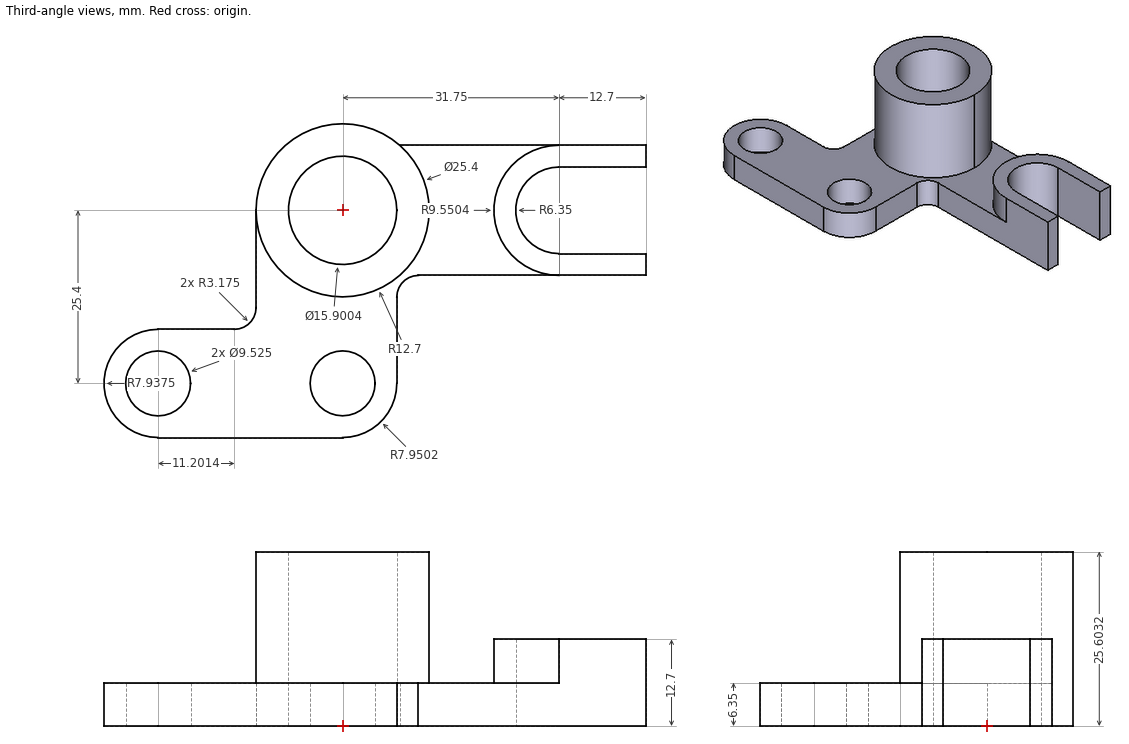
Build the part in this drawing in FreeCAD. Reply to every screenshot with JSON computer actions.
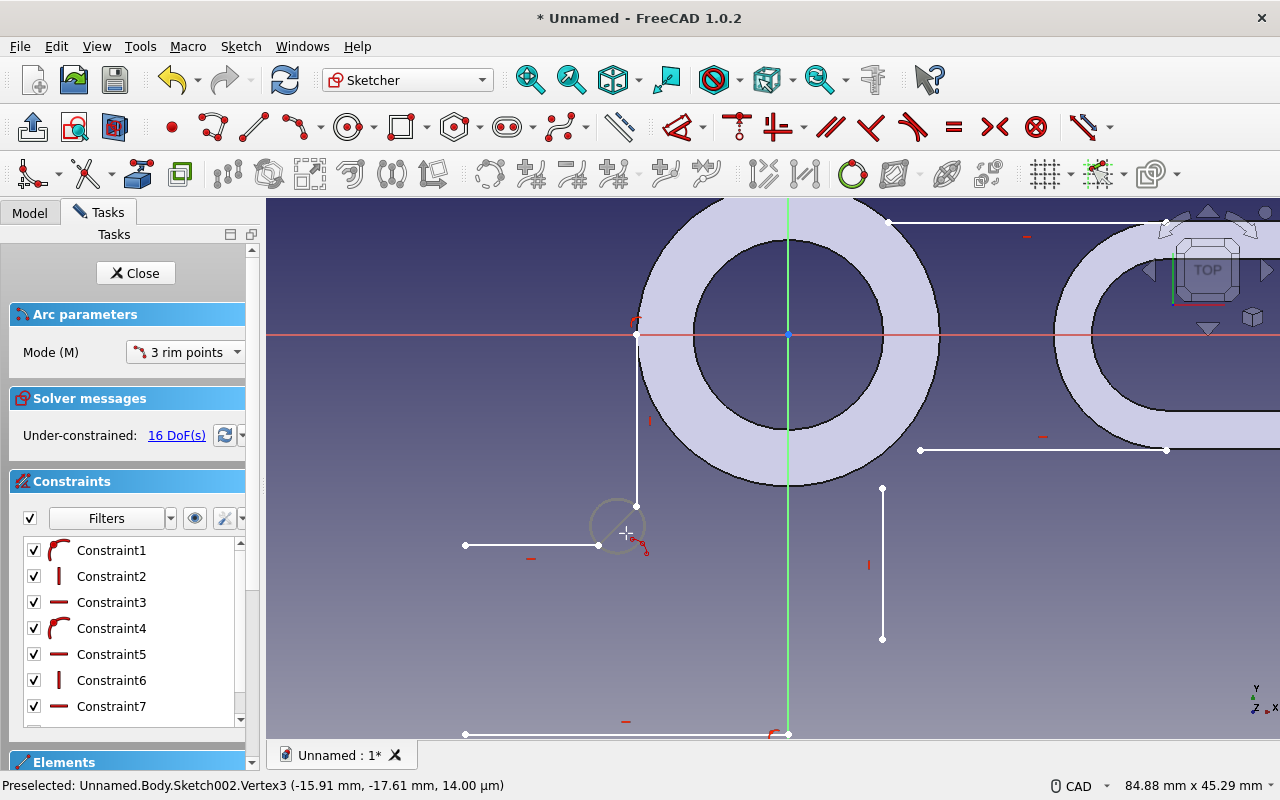
{"action": "left_click", "coordinate": [625, 532]}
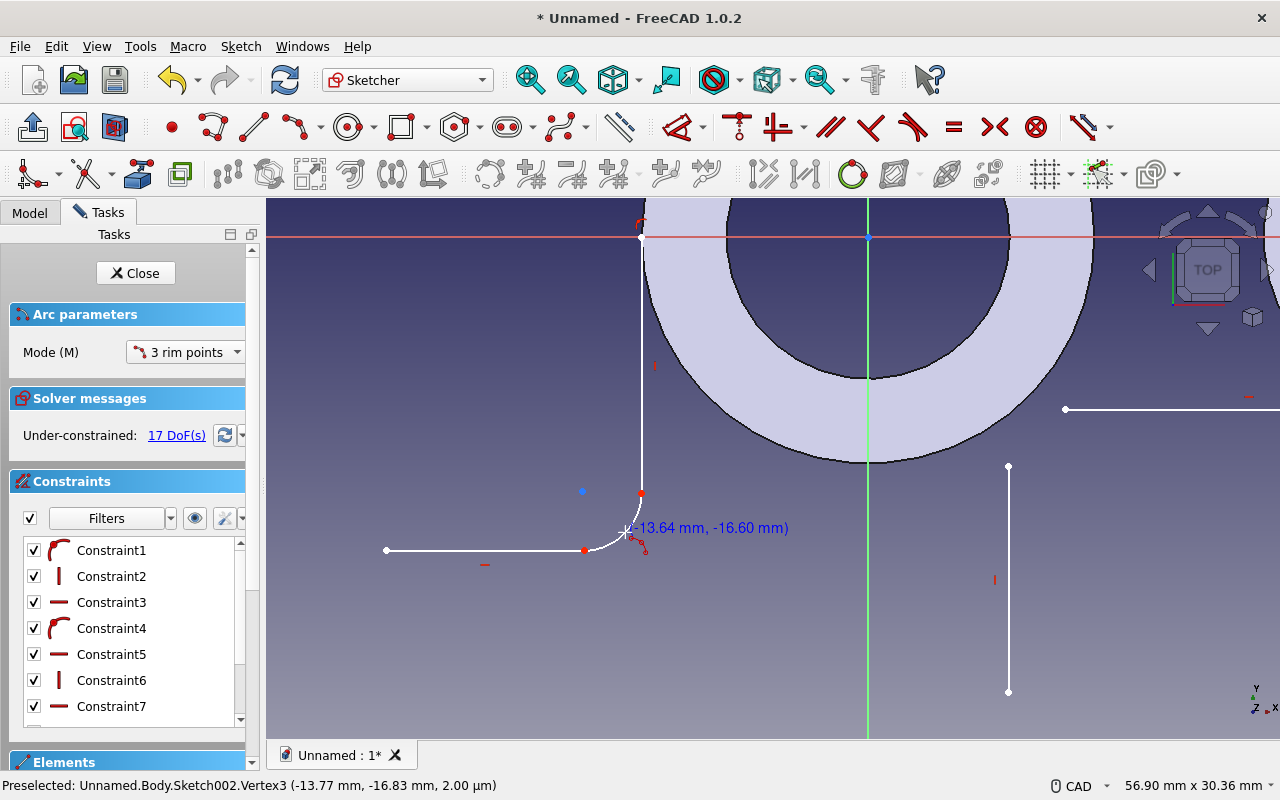
{"action": "left_click", "coordinate": [386, 551]}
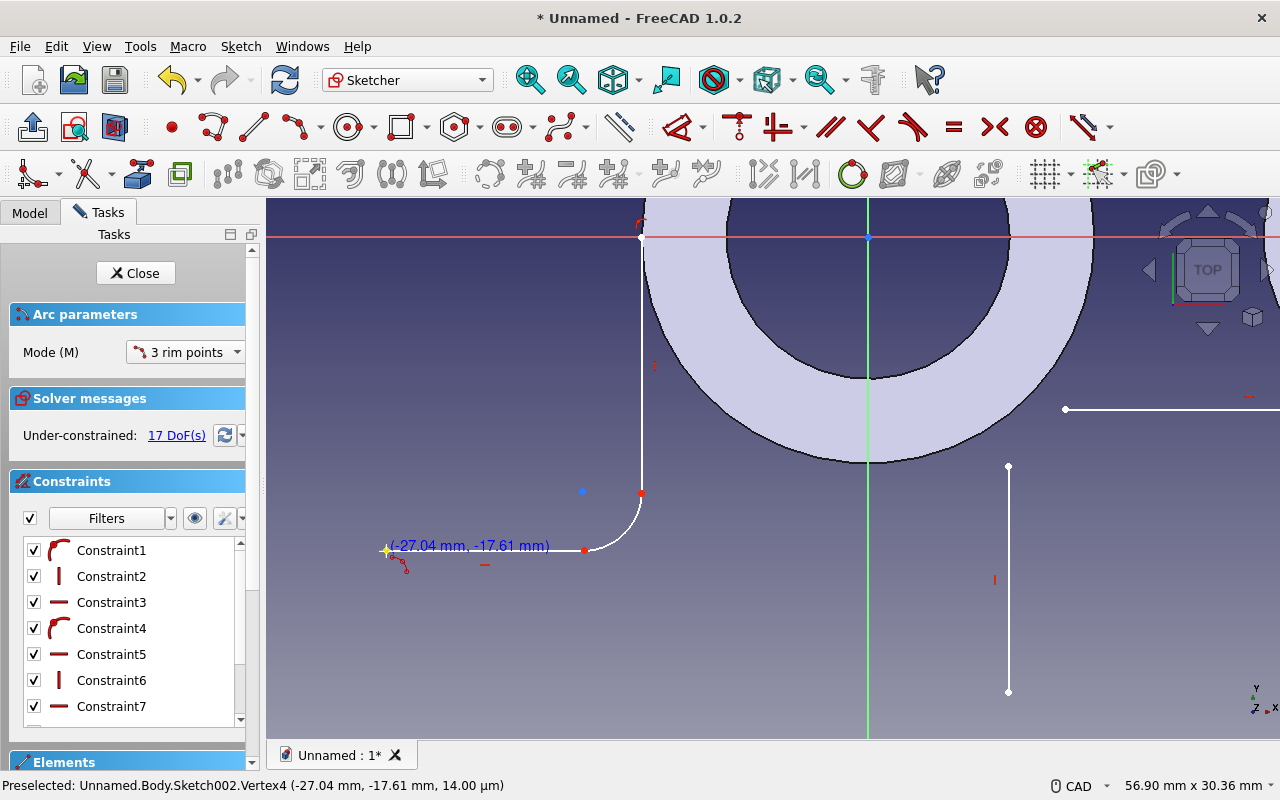
{"action": "scroll", "coordinate": [595, 484], "scroll_direction": "down", "scroll_amount": 4}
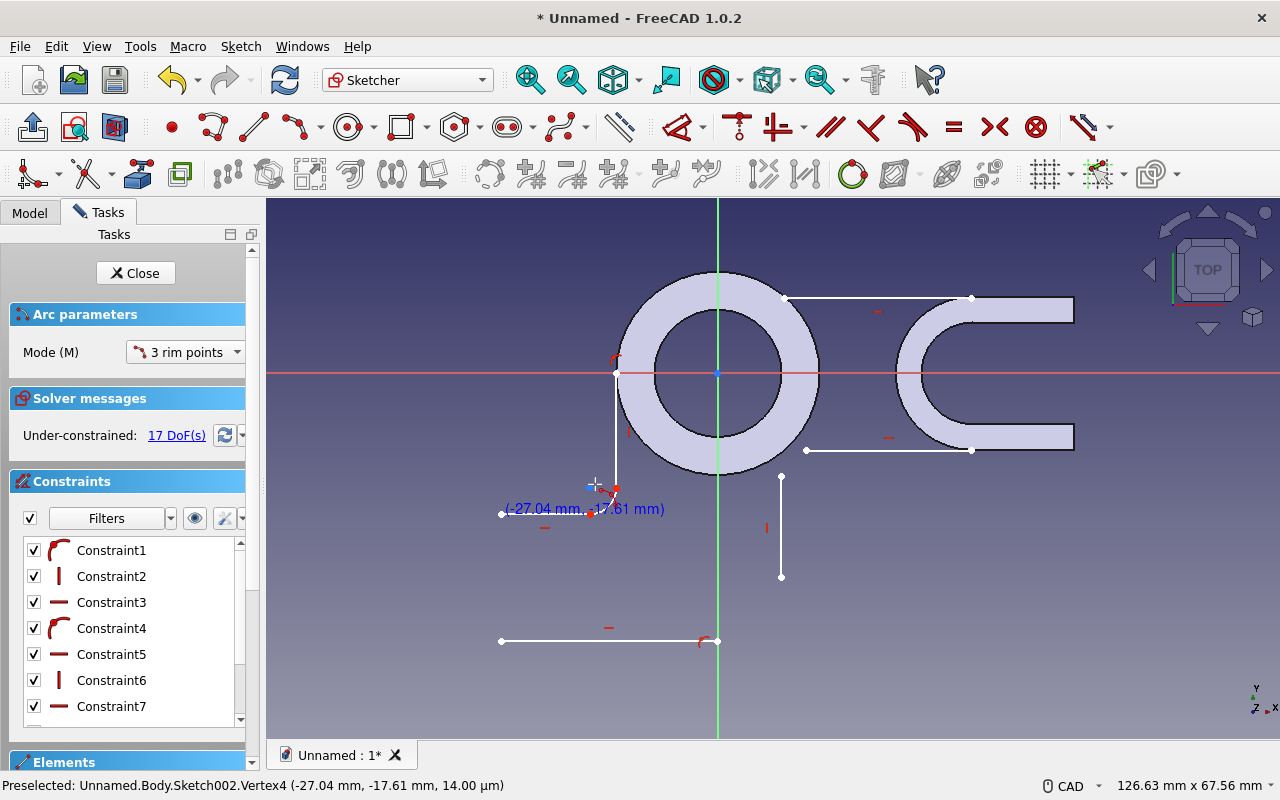
{"action": "left_click", "coordinate": [501, 641]}
{"action": "left_click", "coordinate": [437, 577]}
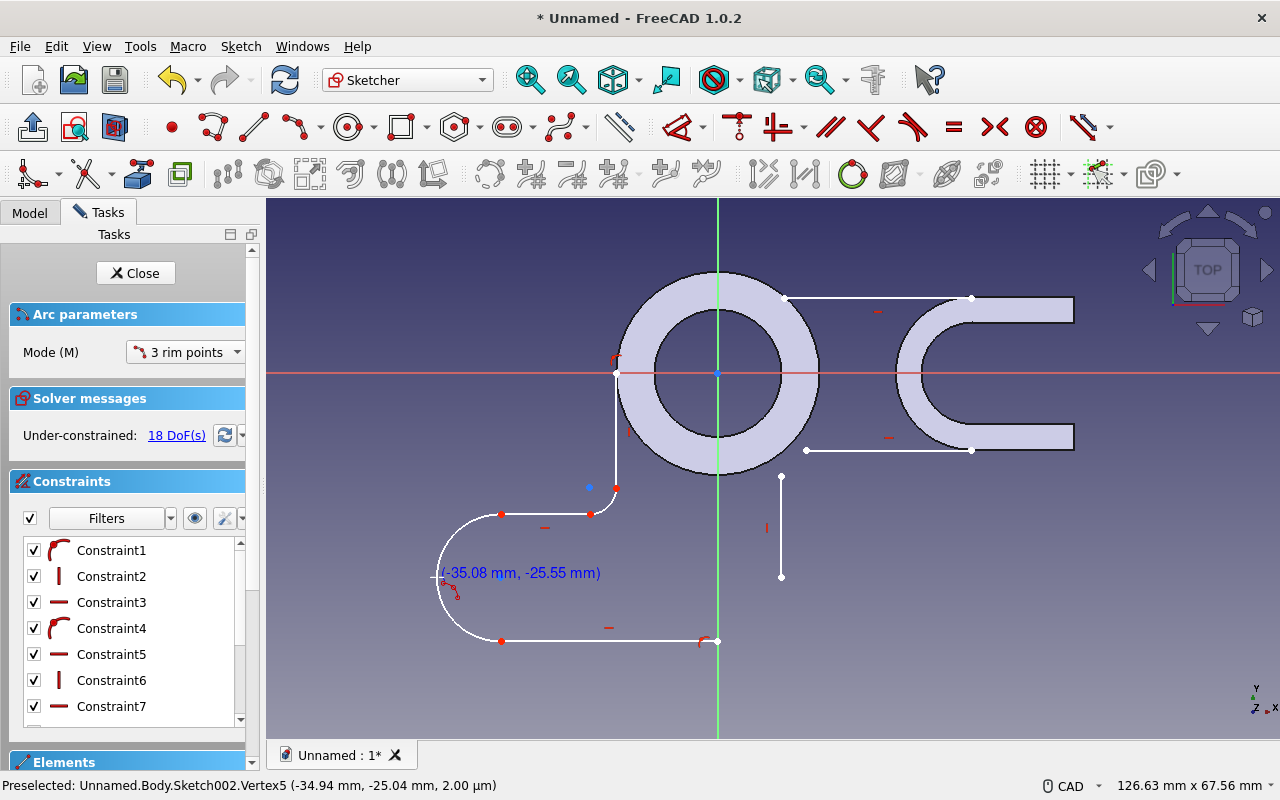
{"action": "left_click", "coordinate": [718, 641]}
{"action": "left_click", "coordinate": [781, 578]}
{"action": "left_click", "coordinate": [763, 622]}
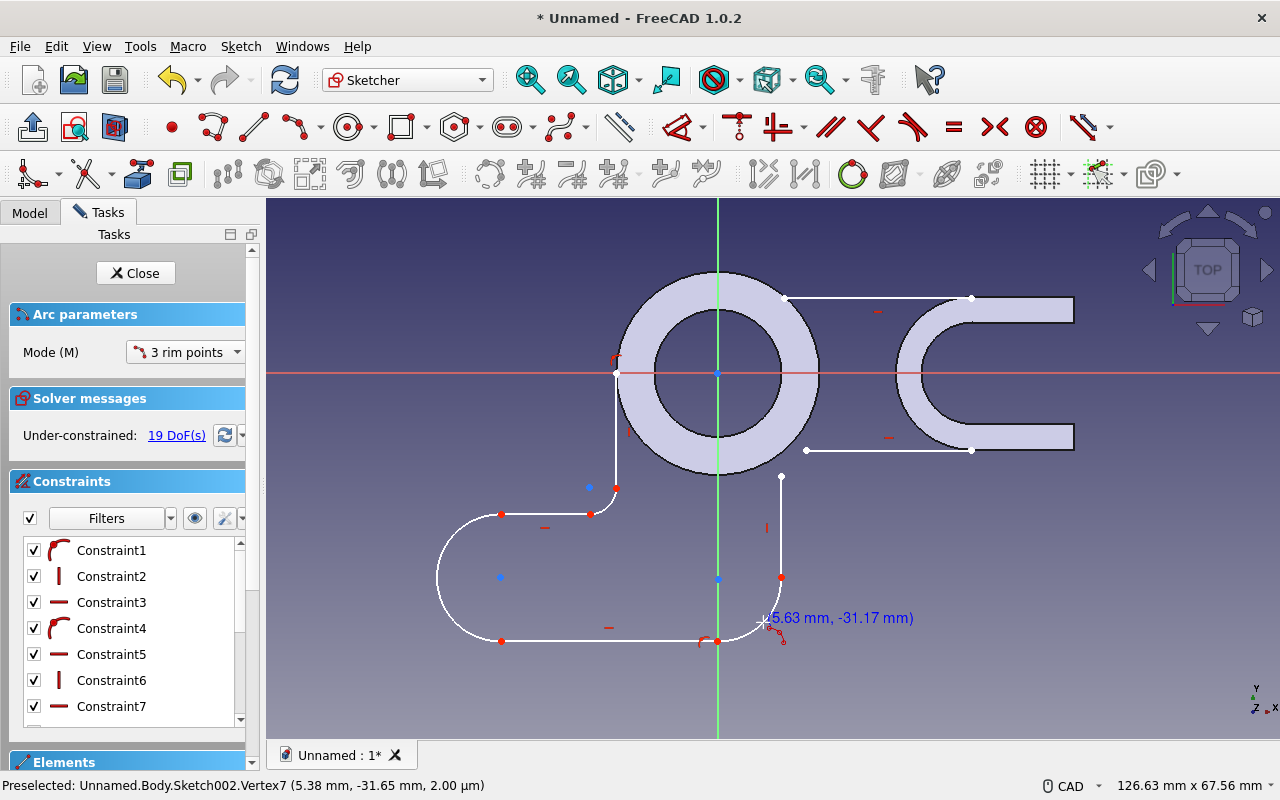
{"action": "left_click", "coordinate": [781, 477]}
{"action": "left_click", "coordinate": [807, 451]}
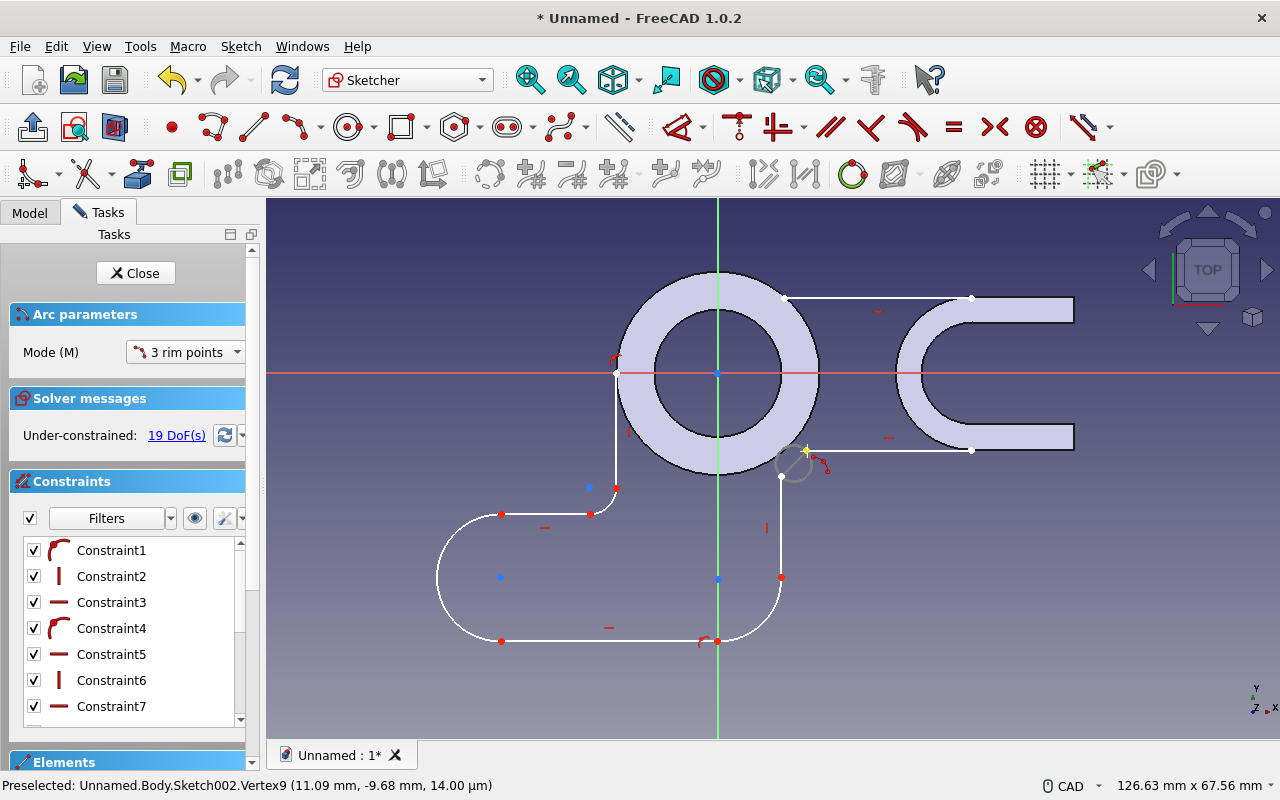
{"action": "scroll", "coordinate": [789, 457], "scroll_direction": "up", "scroll_amount": 4}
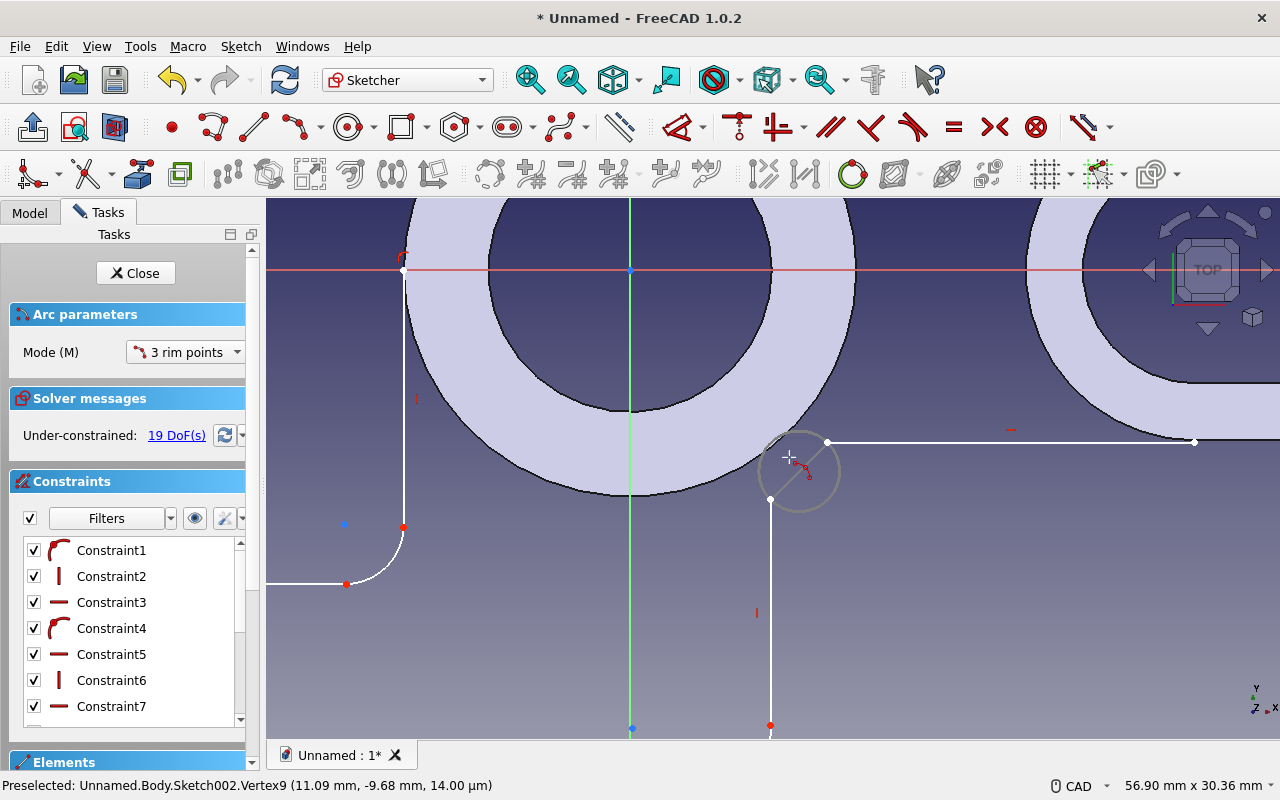
{"action": "left_click", "coordinate": [788, 457]}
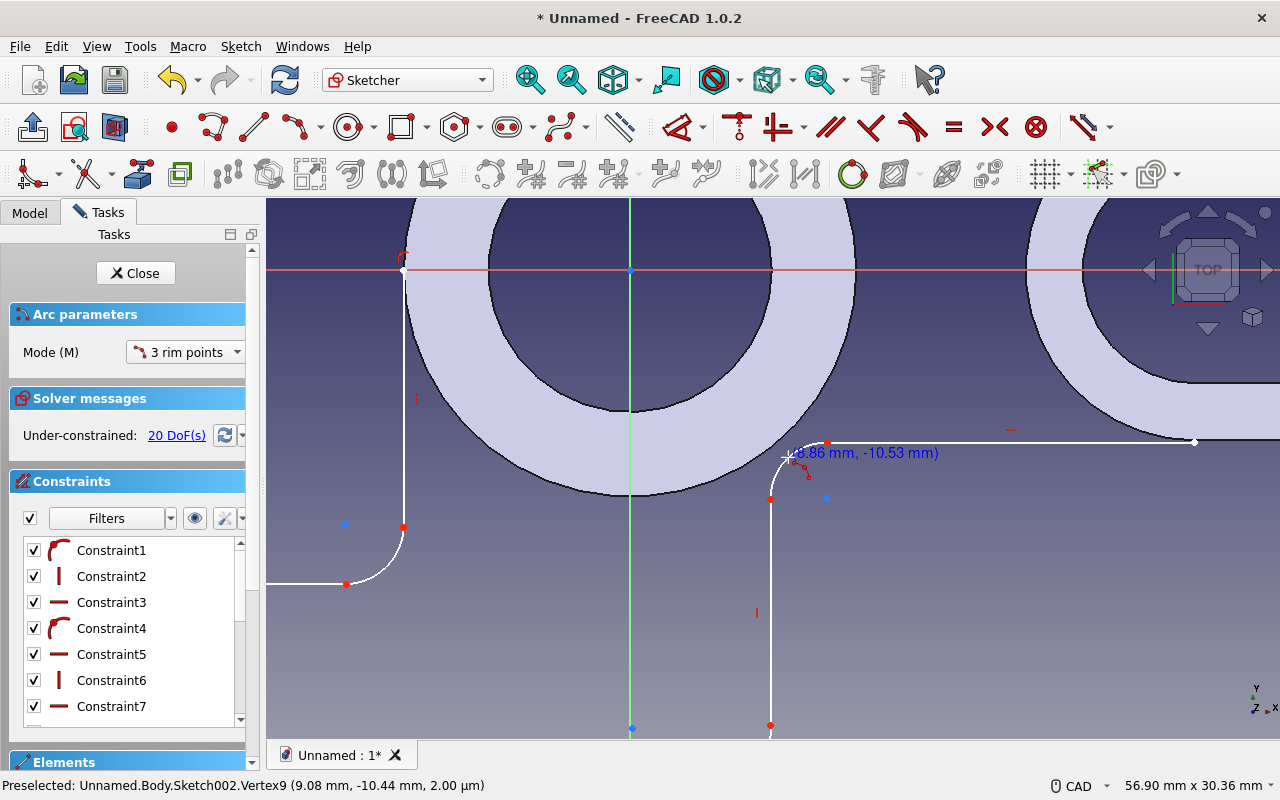
{"action": "scroll", "coordinate": [789, 457], "scroll_direction": "down", "scroll_amount": 4}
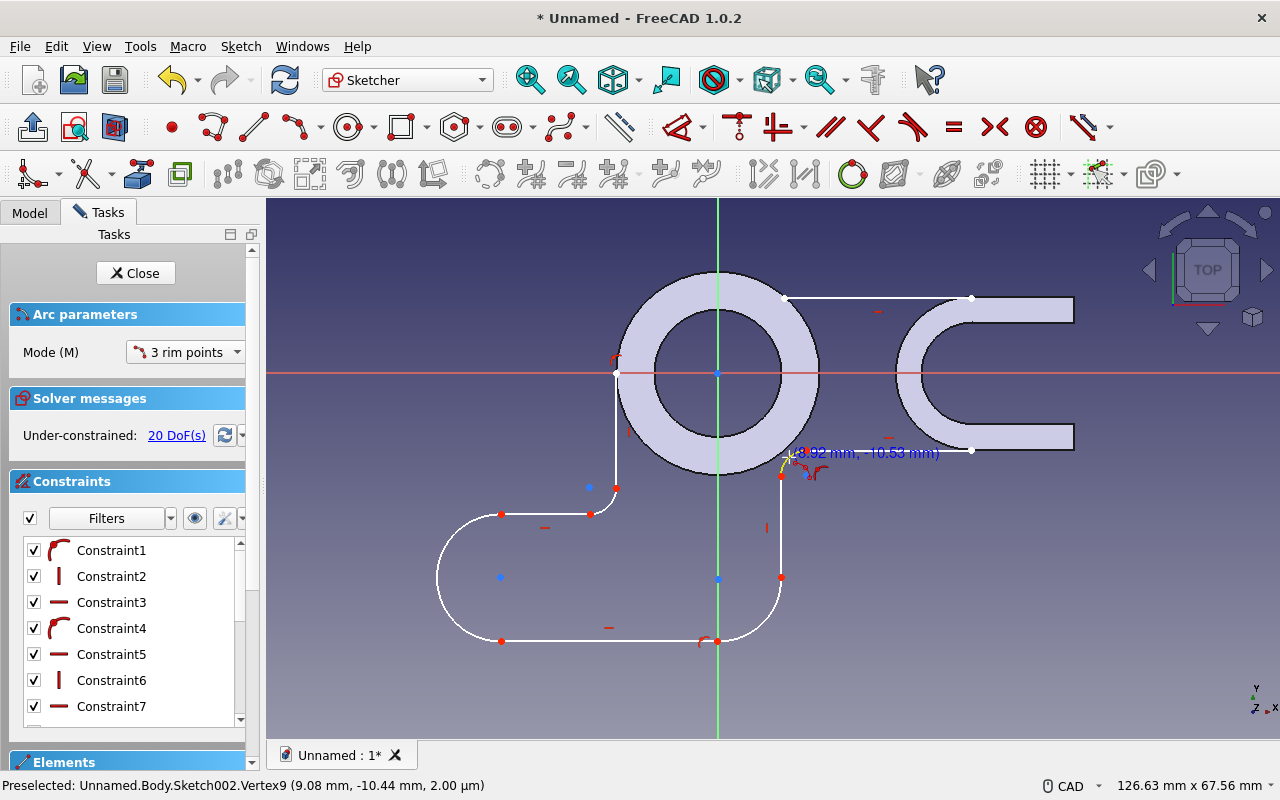
{"action": "left_click", "coordinate": [972, 451]}
{"action": "left_click", "coordinate": [972, 298]}
{"action": "left_click", "coordinate": [899, 350]}